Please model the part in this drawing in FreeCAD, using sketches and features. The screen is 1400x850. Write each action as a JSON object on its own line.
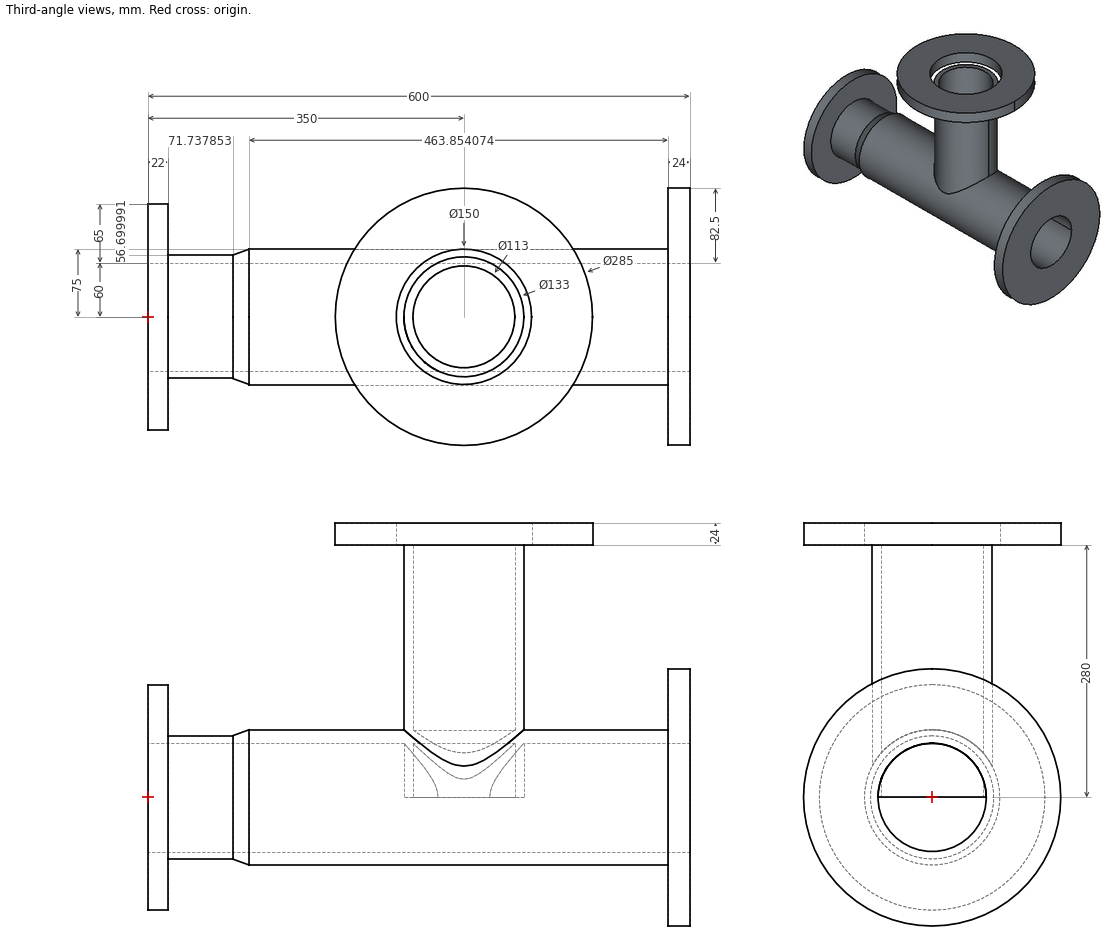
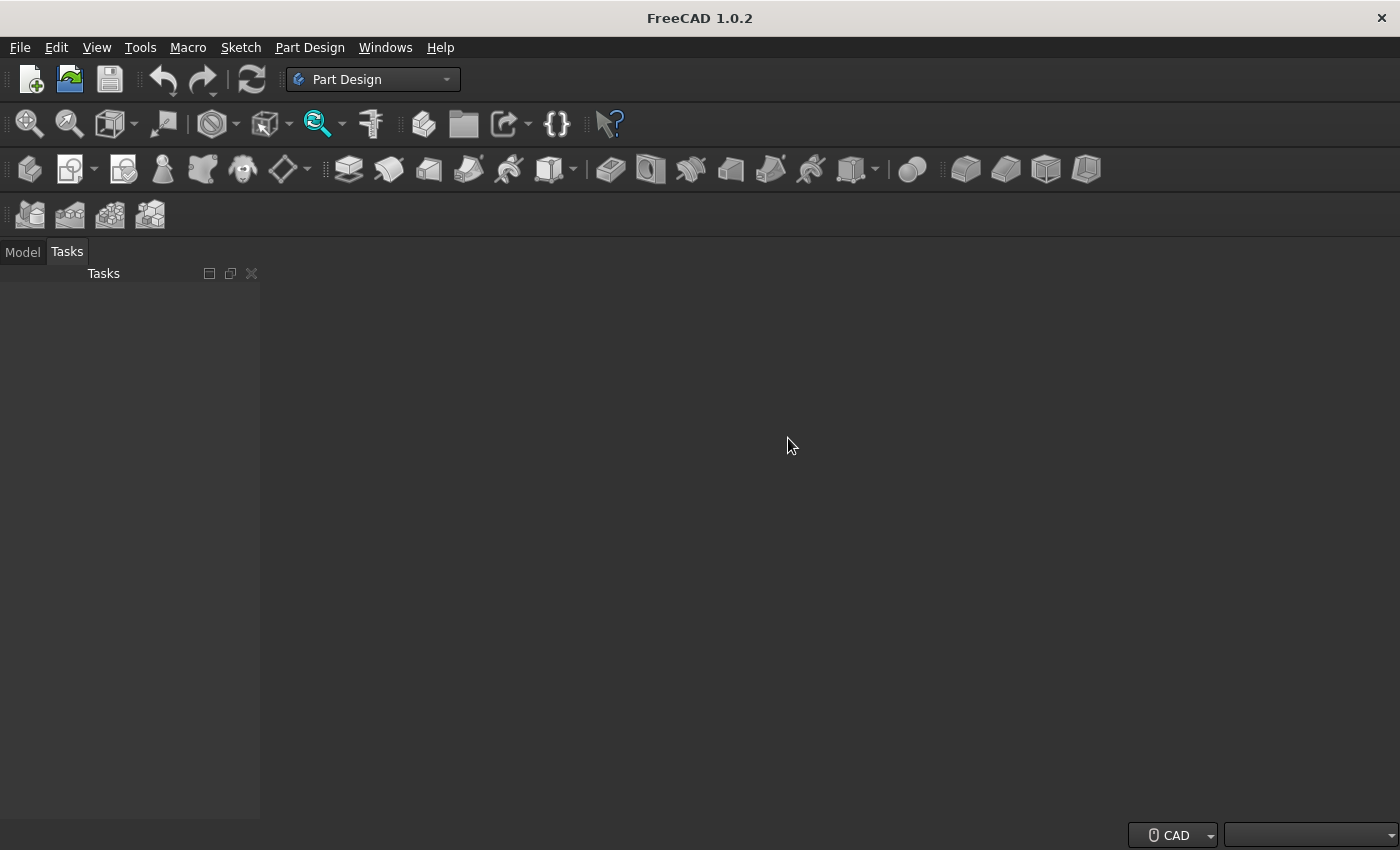
{"action": "left_click", "coordinate": [30, 80]}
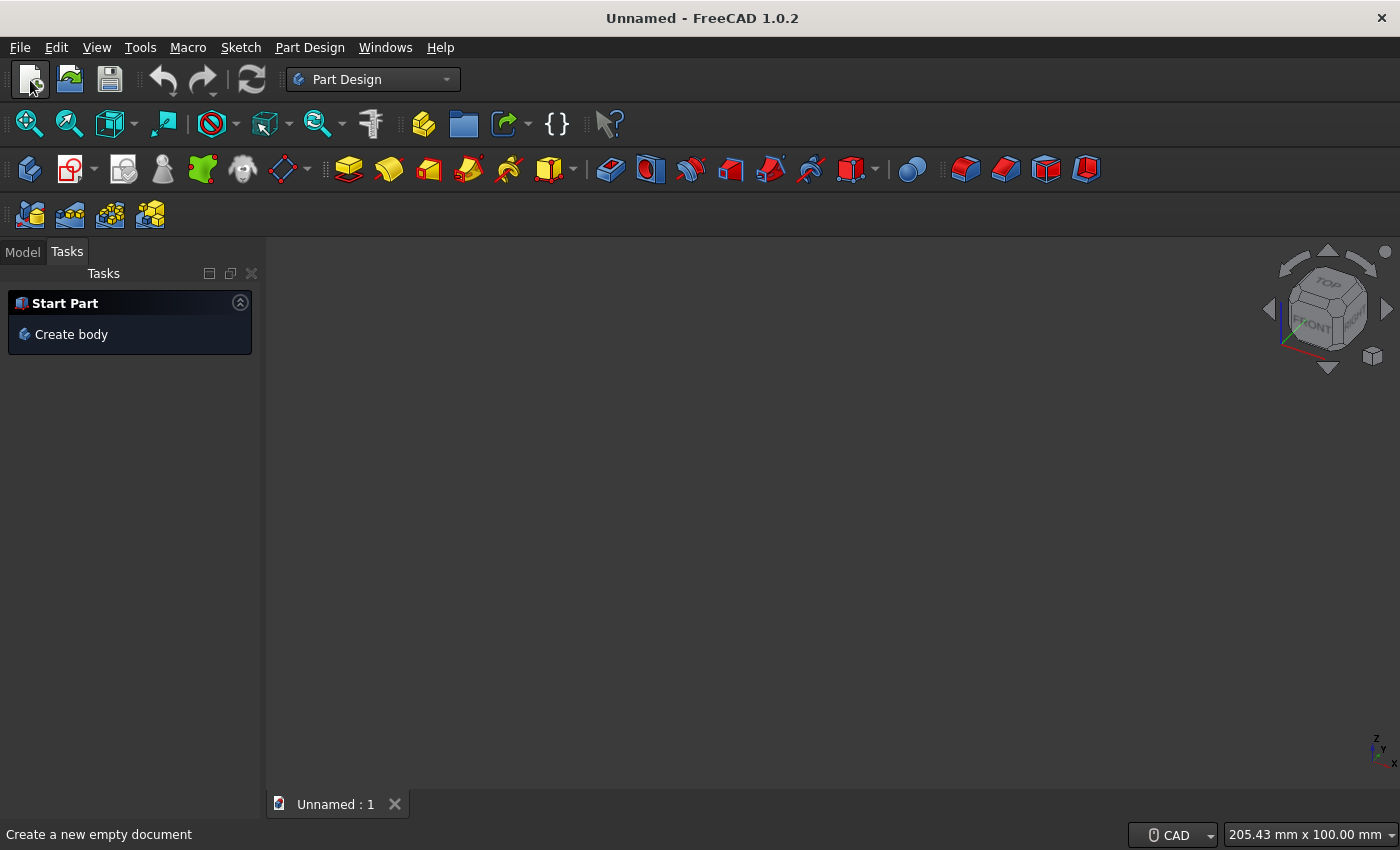
{"action": "left_click", "coordinate": [70, 170]}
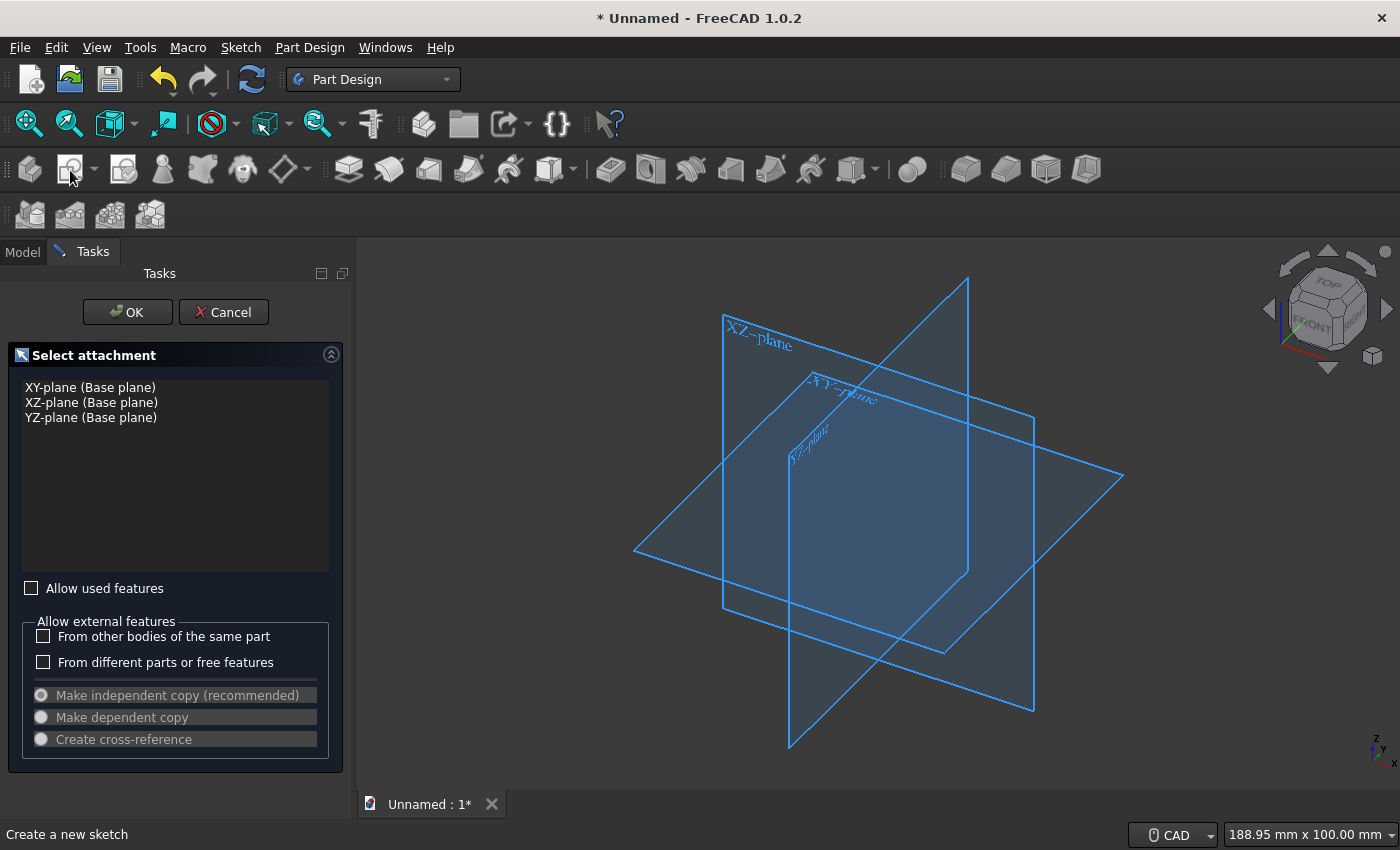
{"action": "left_click", "coordinate": [82, 388]}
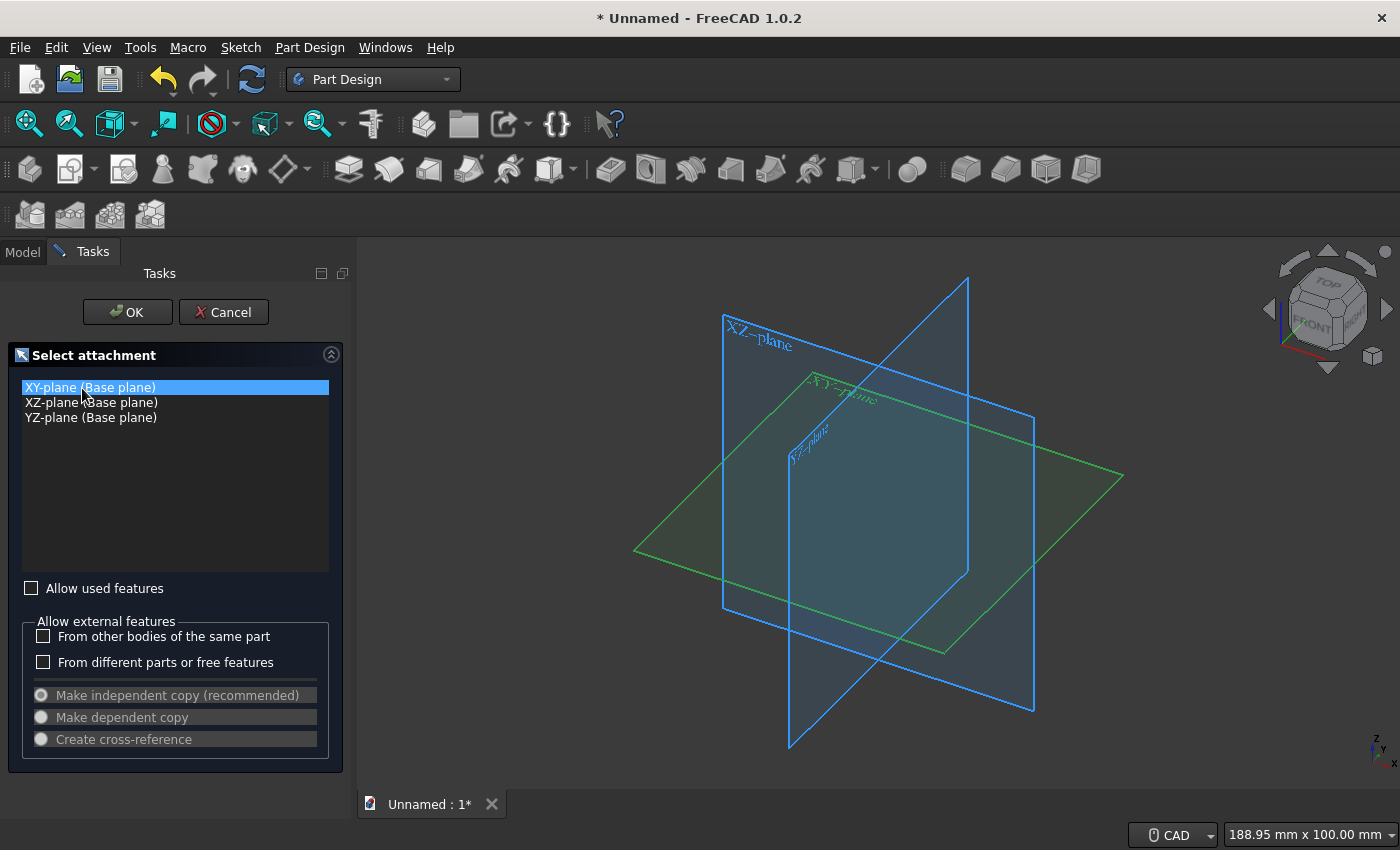
{"action": "left_click", "coordinate": [128, 312]}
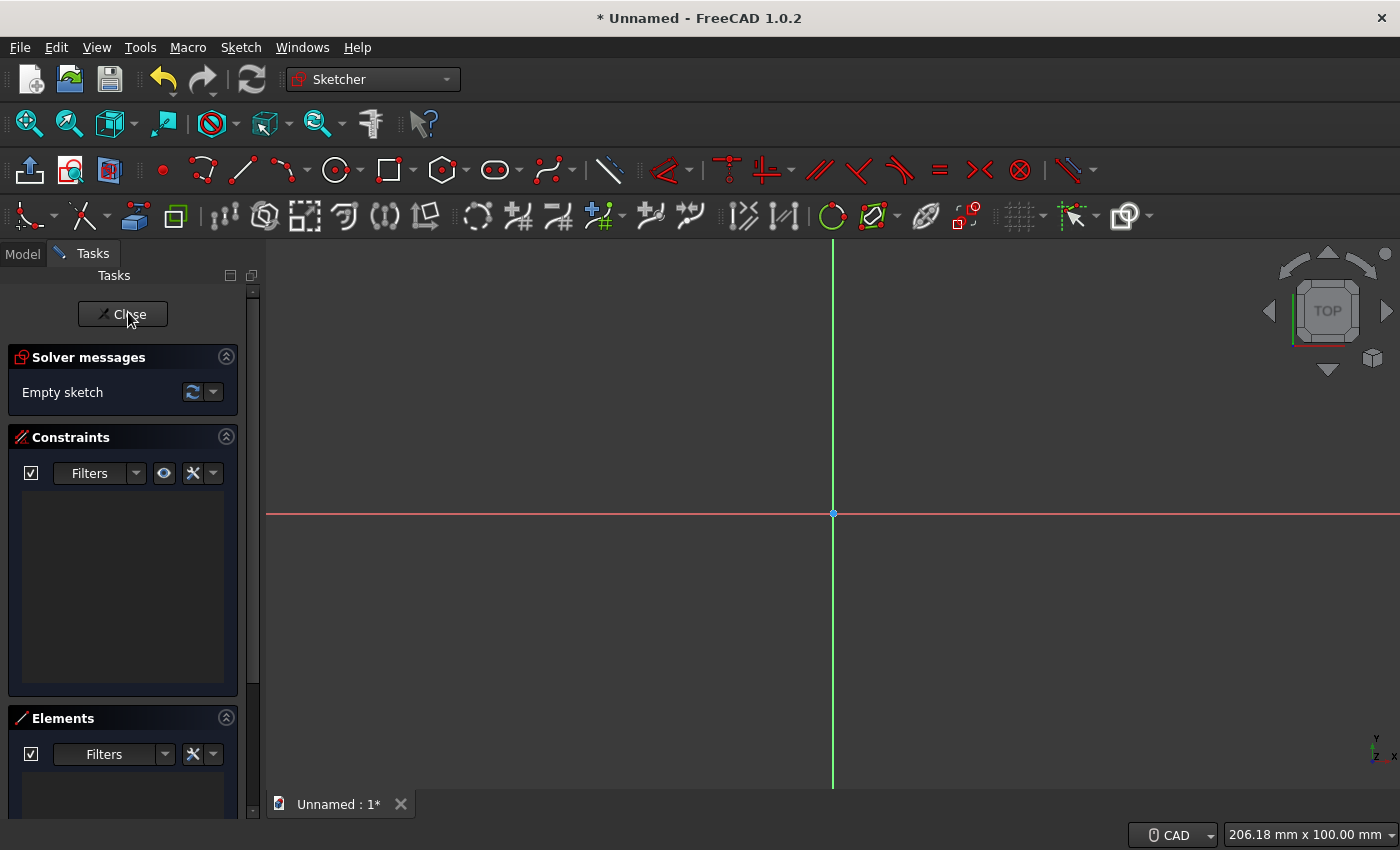
{"action": "scroll", "coordinate": [330, 613], "scroll_direction": "down", "scroll_amount": 8}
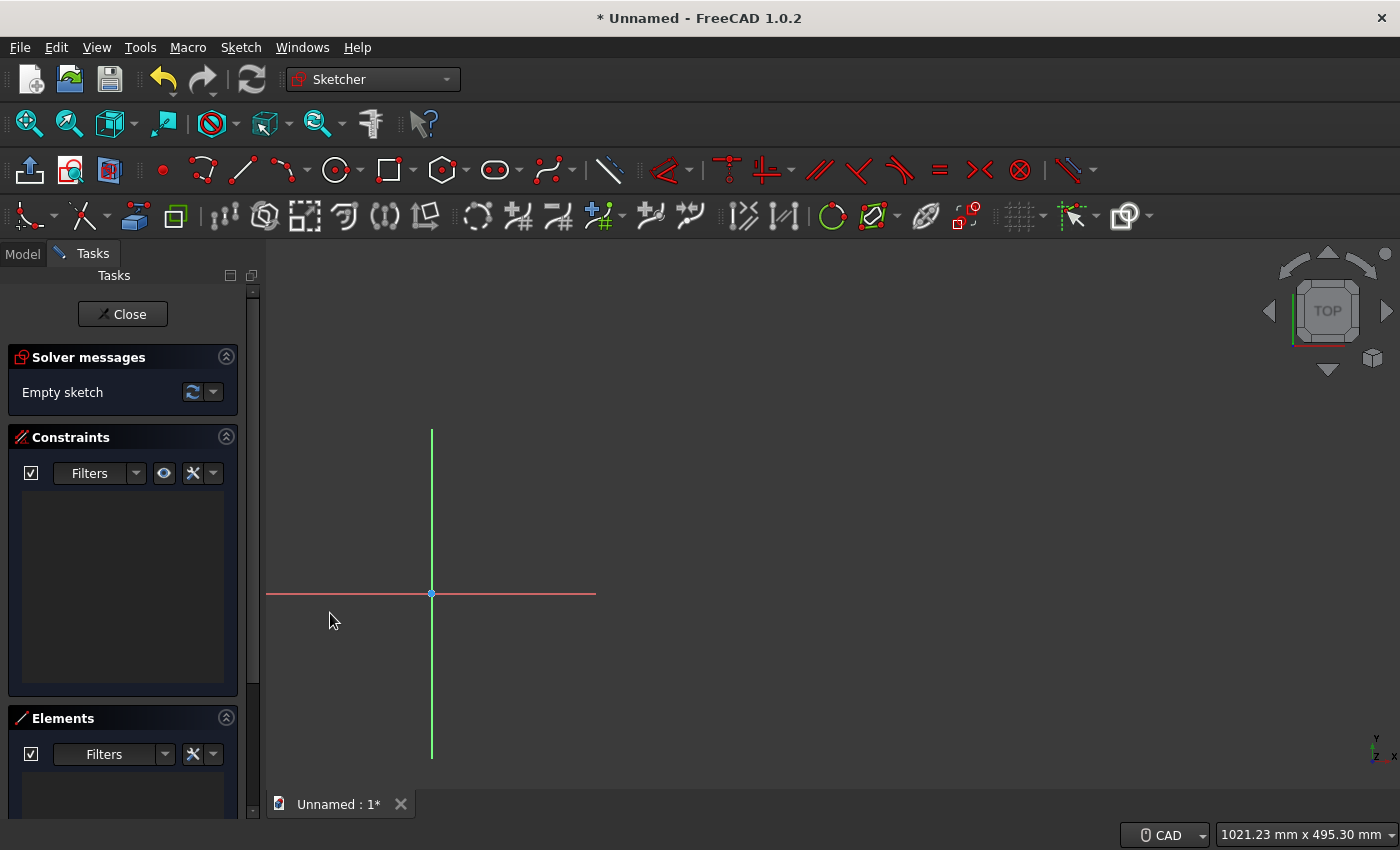
{"action": "key", "text": "g m"}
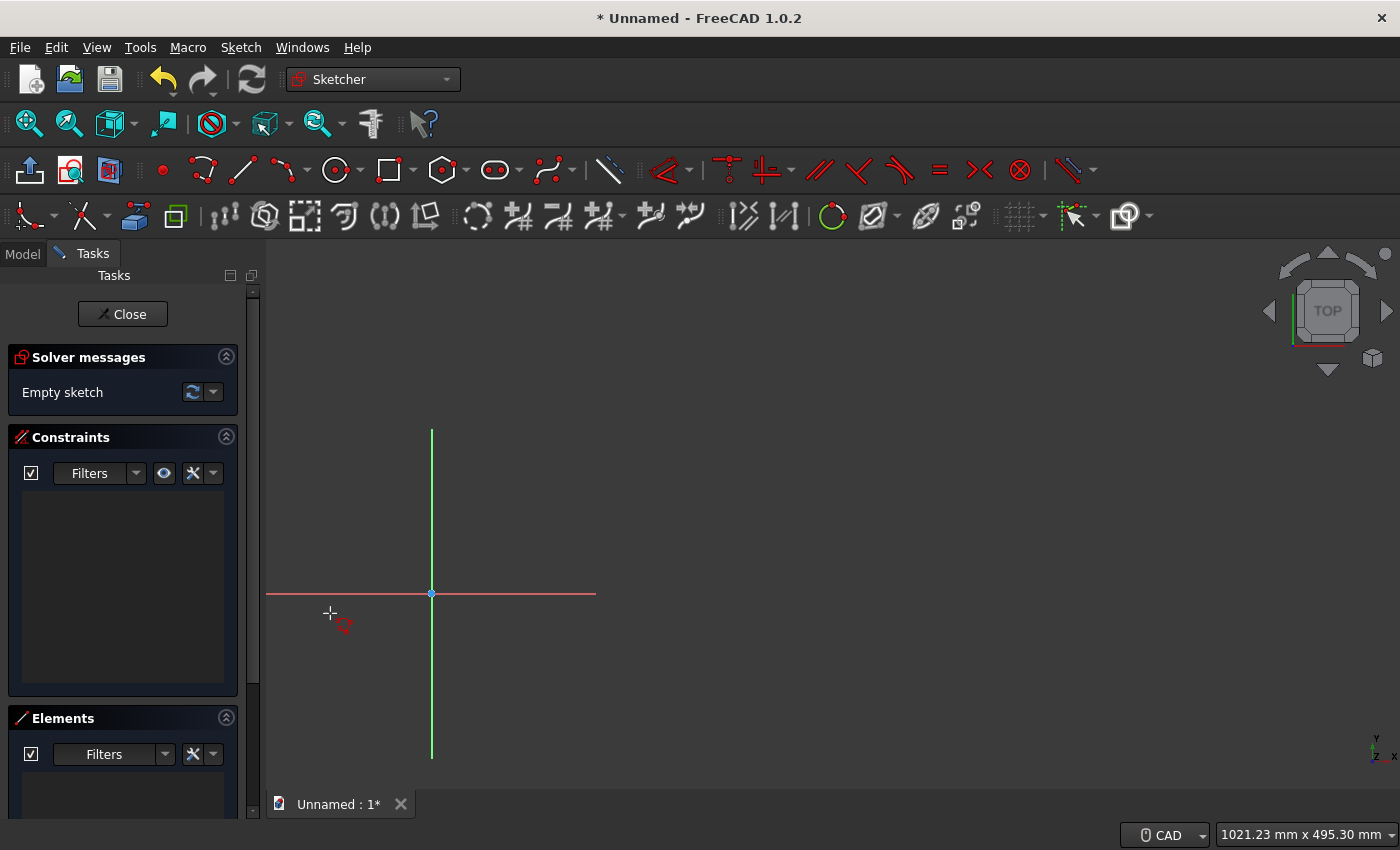
{"action": "left_click", "coordinate": [432, 527]}
{"action": "left_click", "coordinate": [1098, 527]}
{"action": "left_click", "coordinate": [1098, 435]}
{"action": "left_click", "coordinate": [1071, 435]}
{"action": "left_click", "coordinate": [1071, 510]}
{"action": "left_click", "coordinate": [556, 510]}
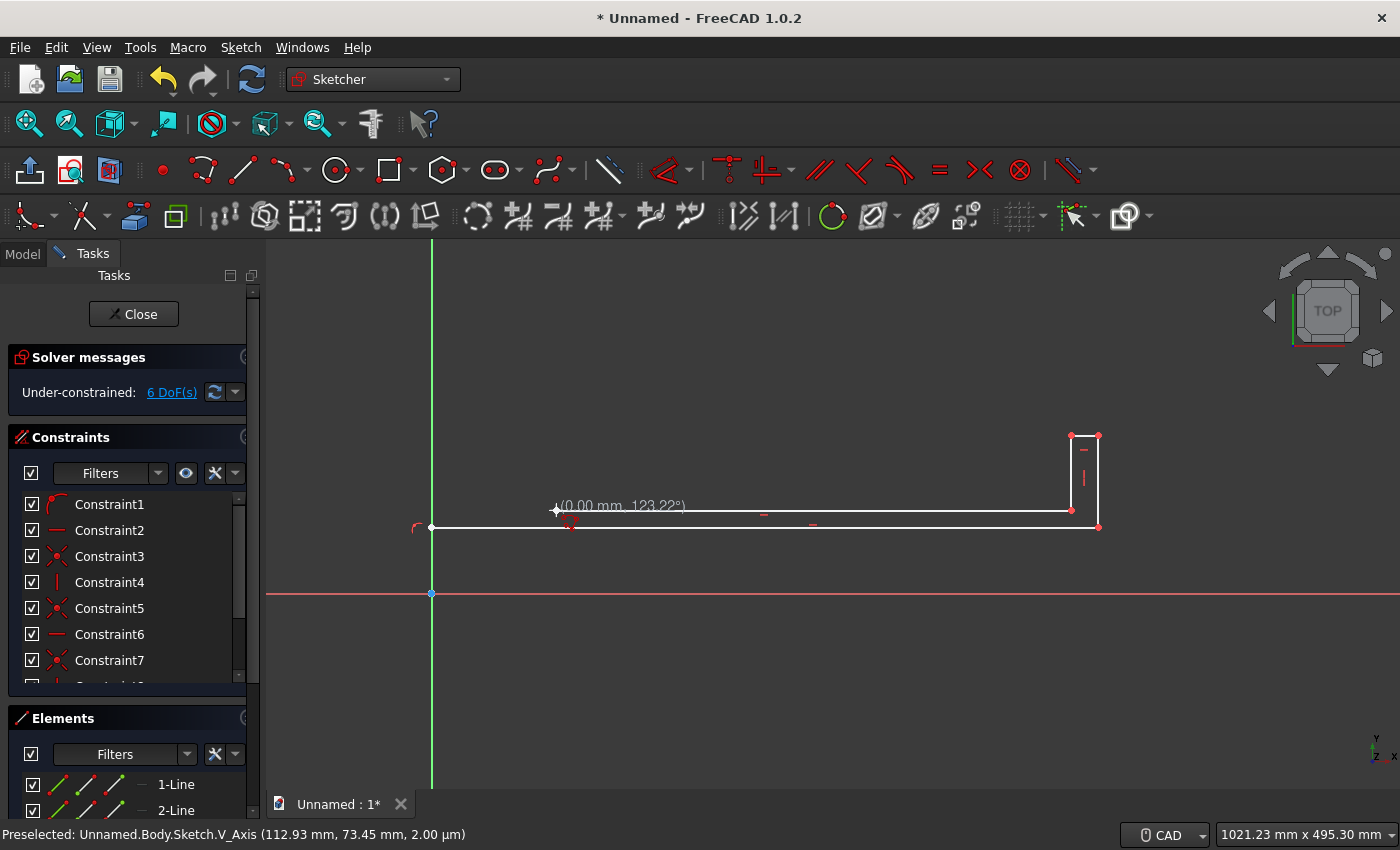
{"action": "scroll", "coordinate": [536, 518], "scroll_direction": "up", "scroll_amount": 3}